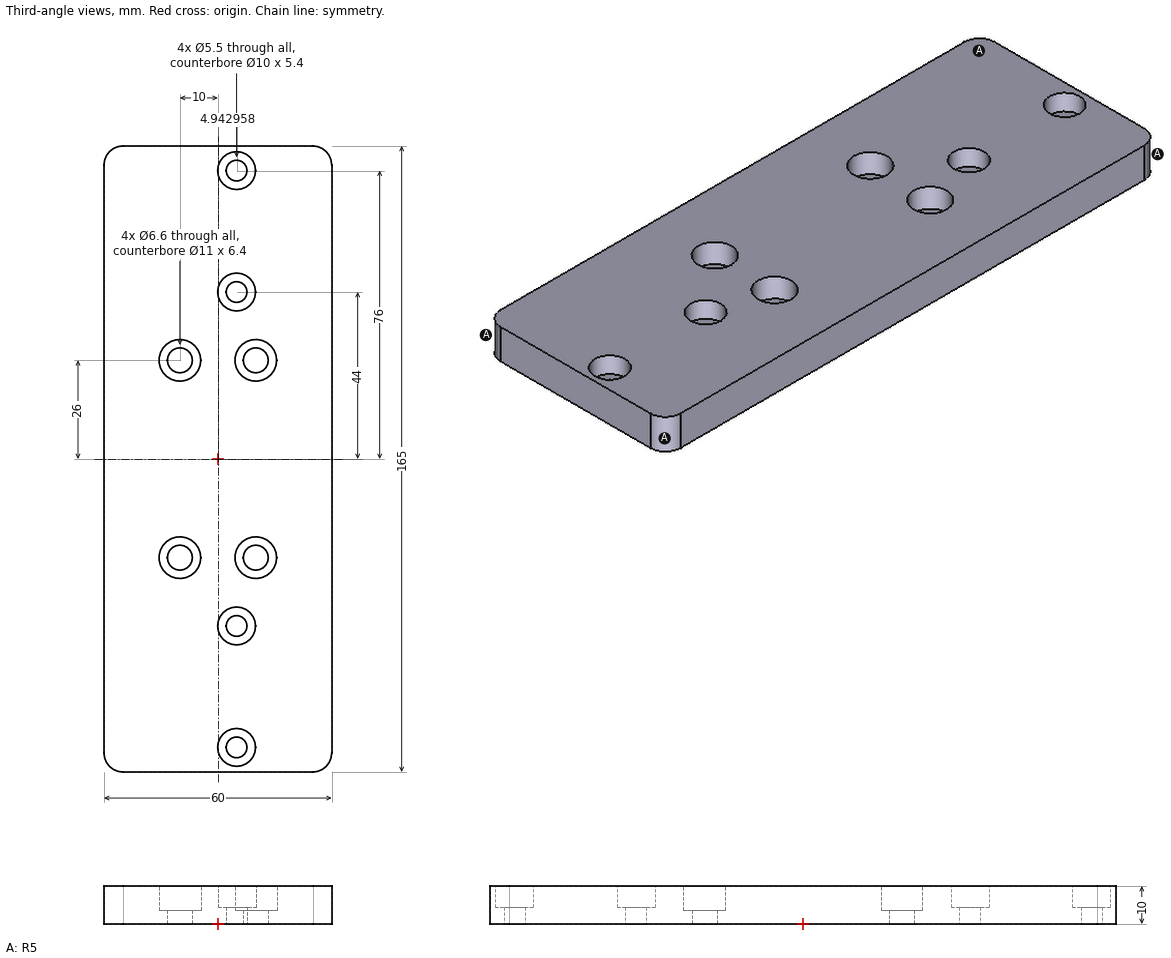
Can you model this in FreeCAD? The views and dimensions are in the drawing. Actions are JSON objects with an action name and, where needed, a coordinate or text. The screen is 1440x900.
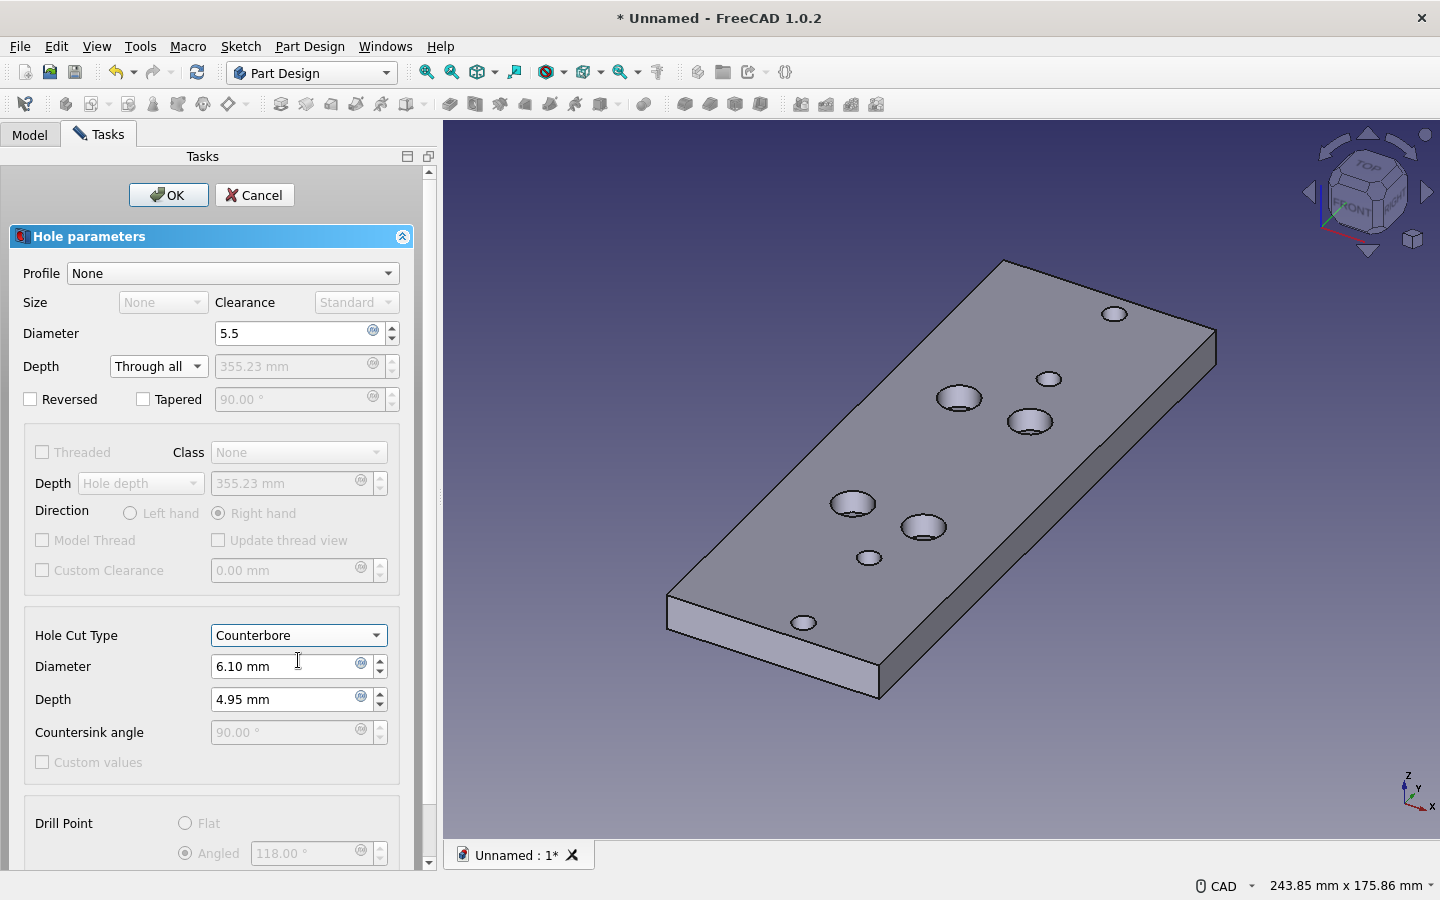
{"action": "triple_click", "coordinate": [292, 666]}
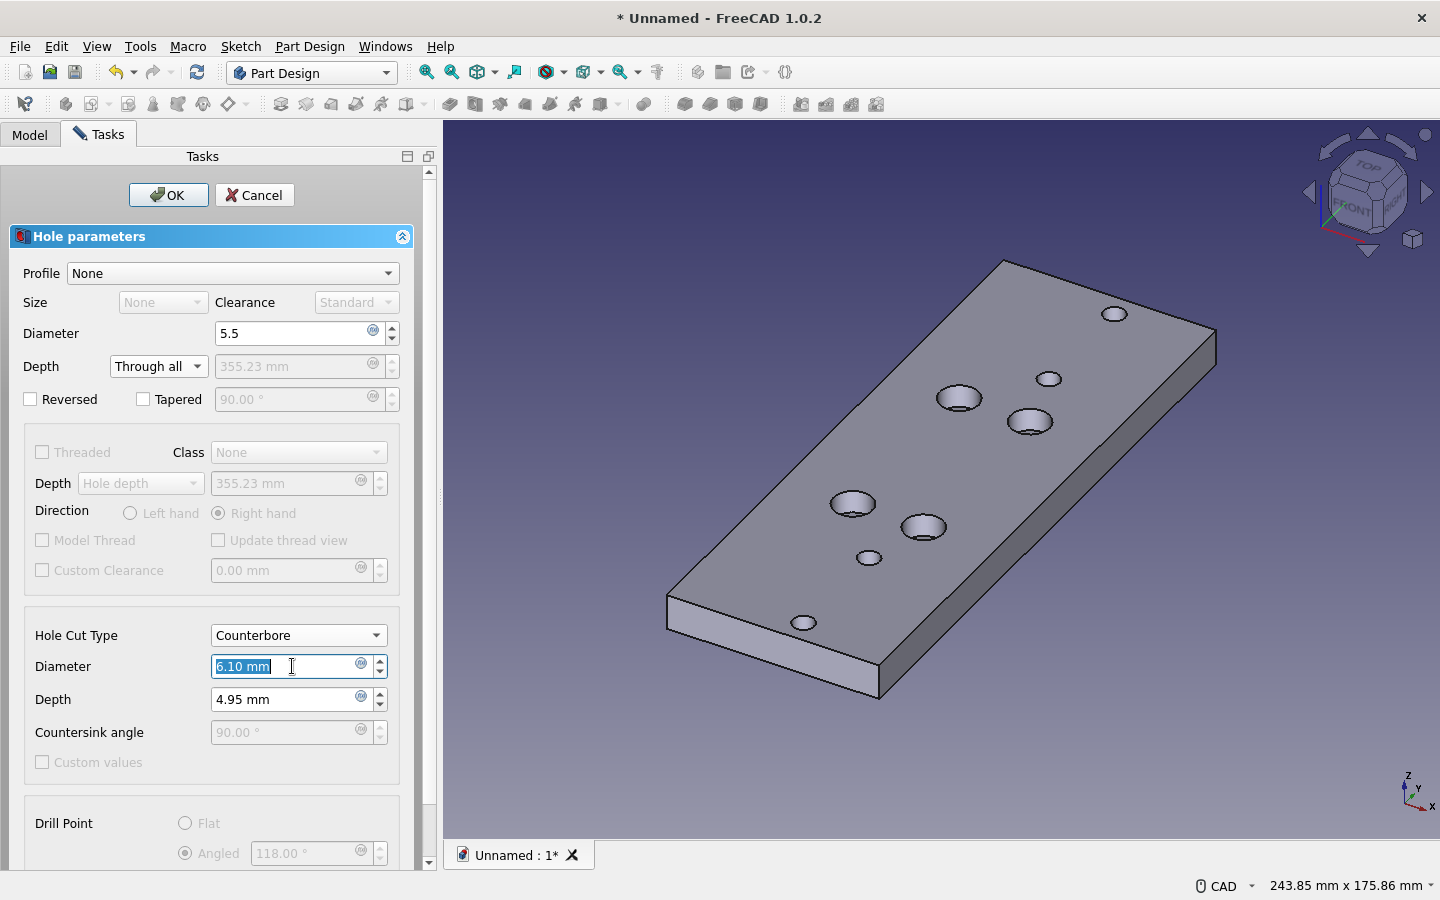
{"action": "type", "text": "10"}
{"action": "key", "text": "Tab"}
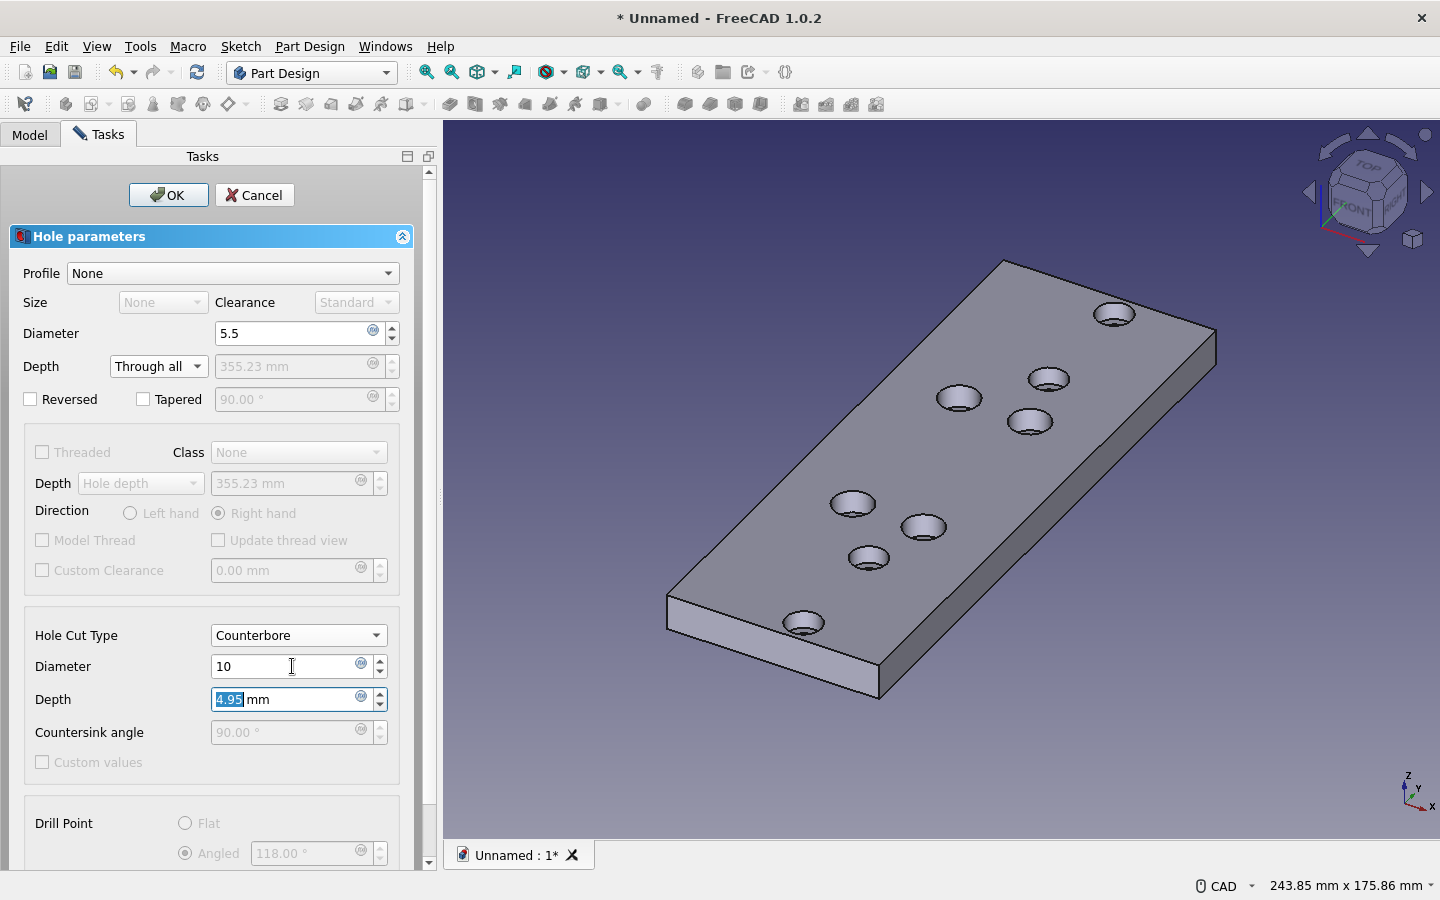
{"action": "type", "text": "5.4"}
{"action": "key", "text": "Tab"}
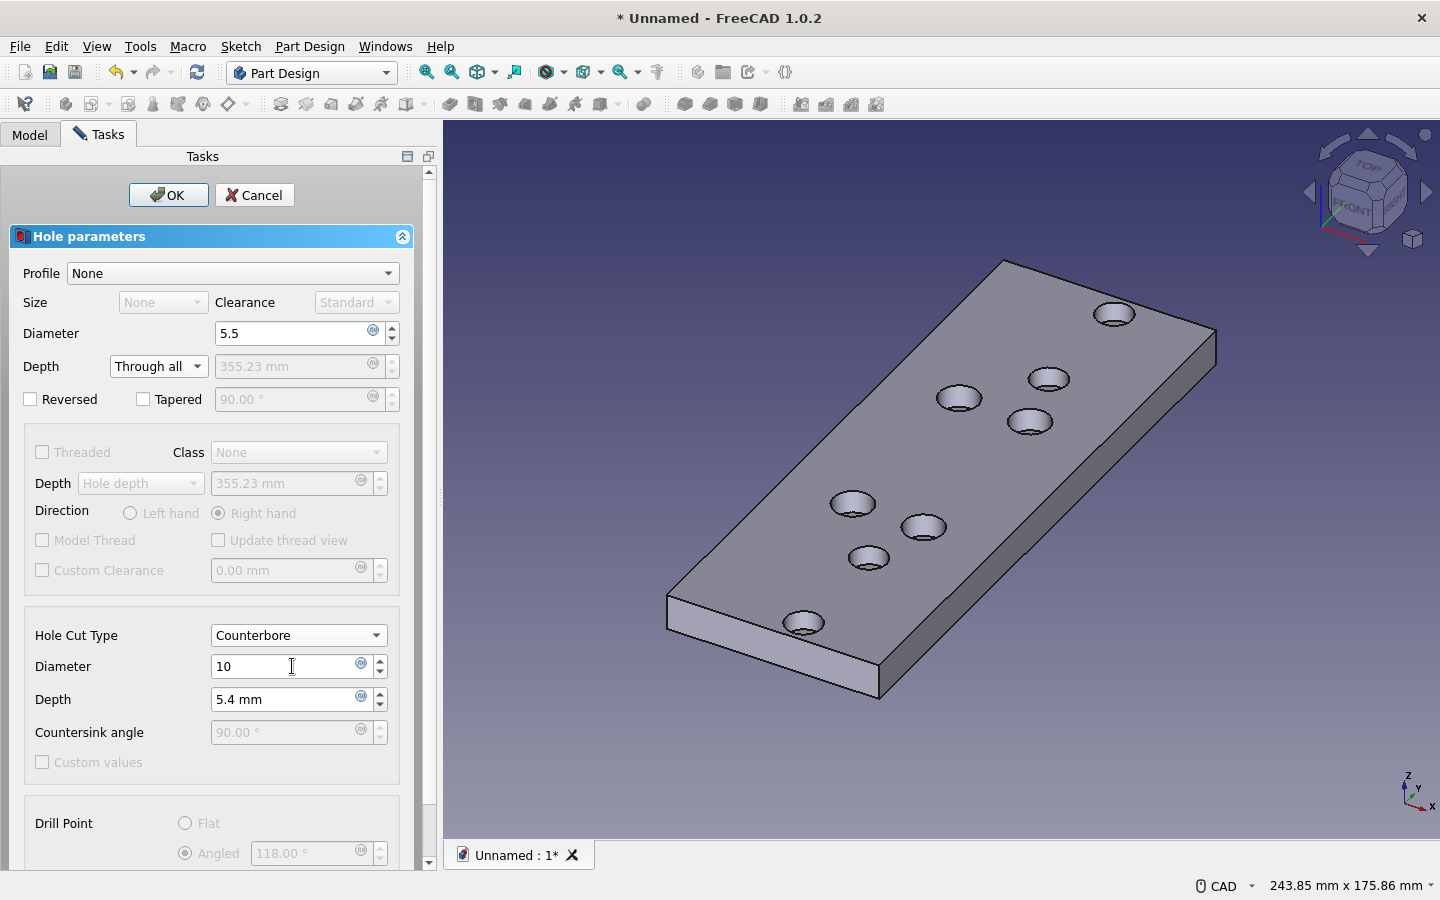
{"action": "left_click", "coordinate": [169, 195]}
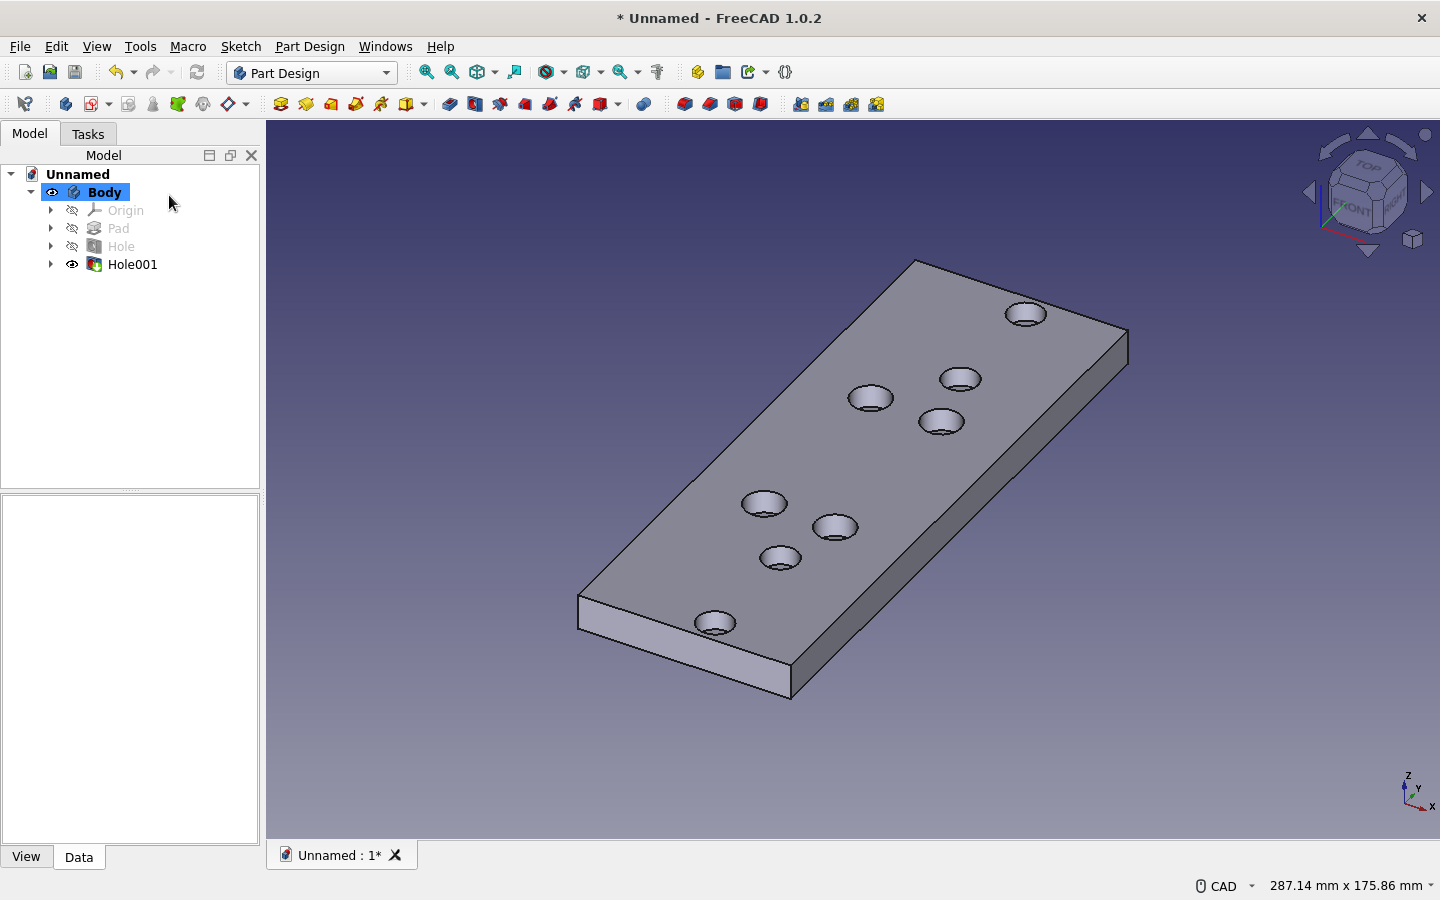
{"action": "left_click", "coordinate": [791, 681]}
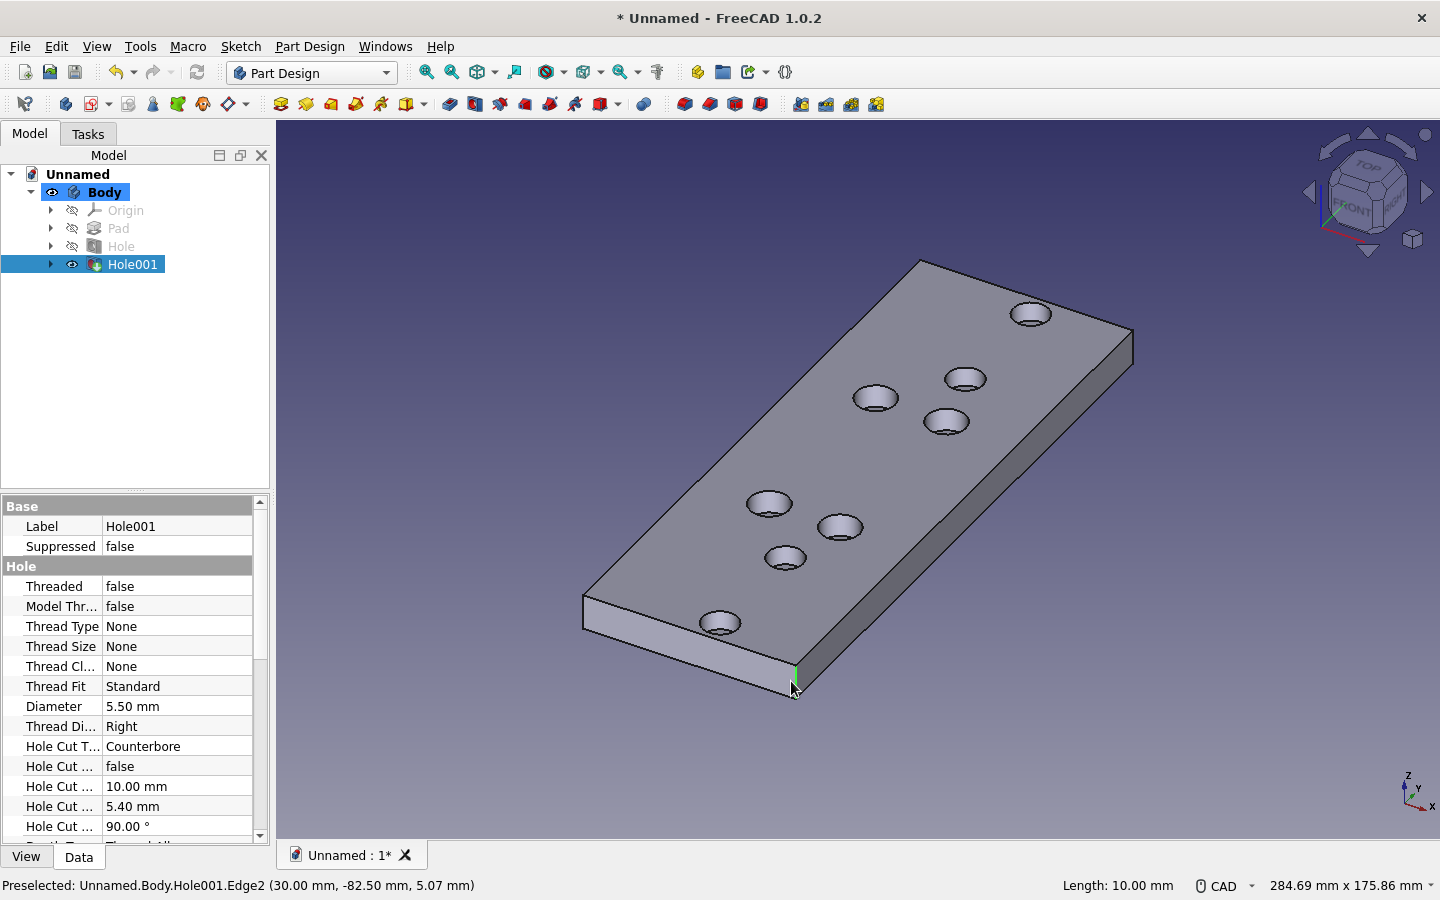
{"action": "key", "text": "0"}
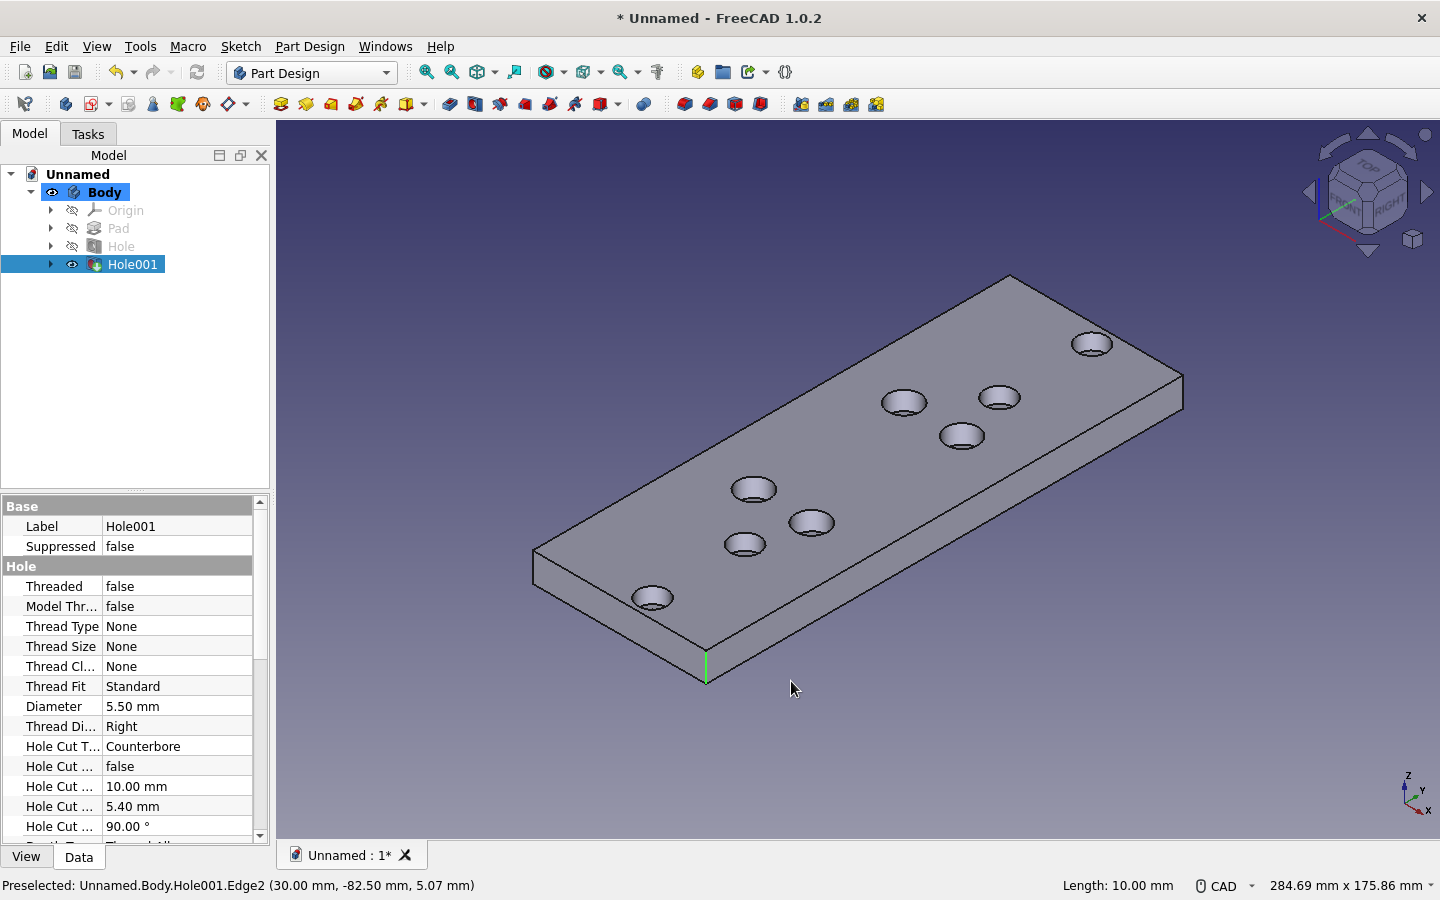
{"action": "key", "text": "2"}